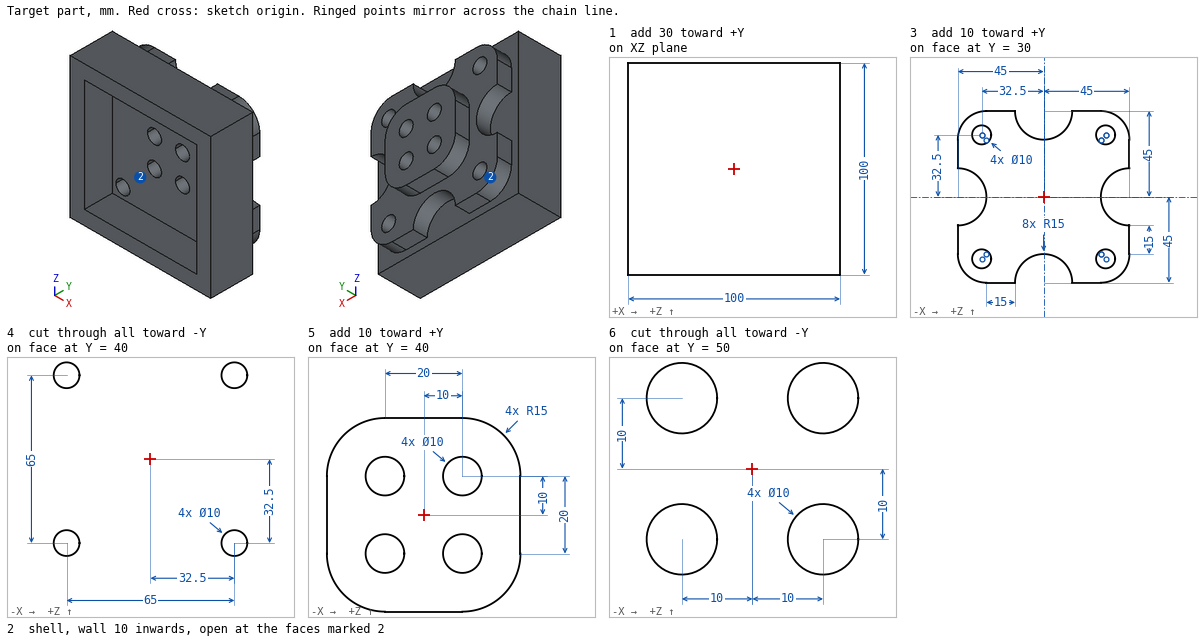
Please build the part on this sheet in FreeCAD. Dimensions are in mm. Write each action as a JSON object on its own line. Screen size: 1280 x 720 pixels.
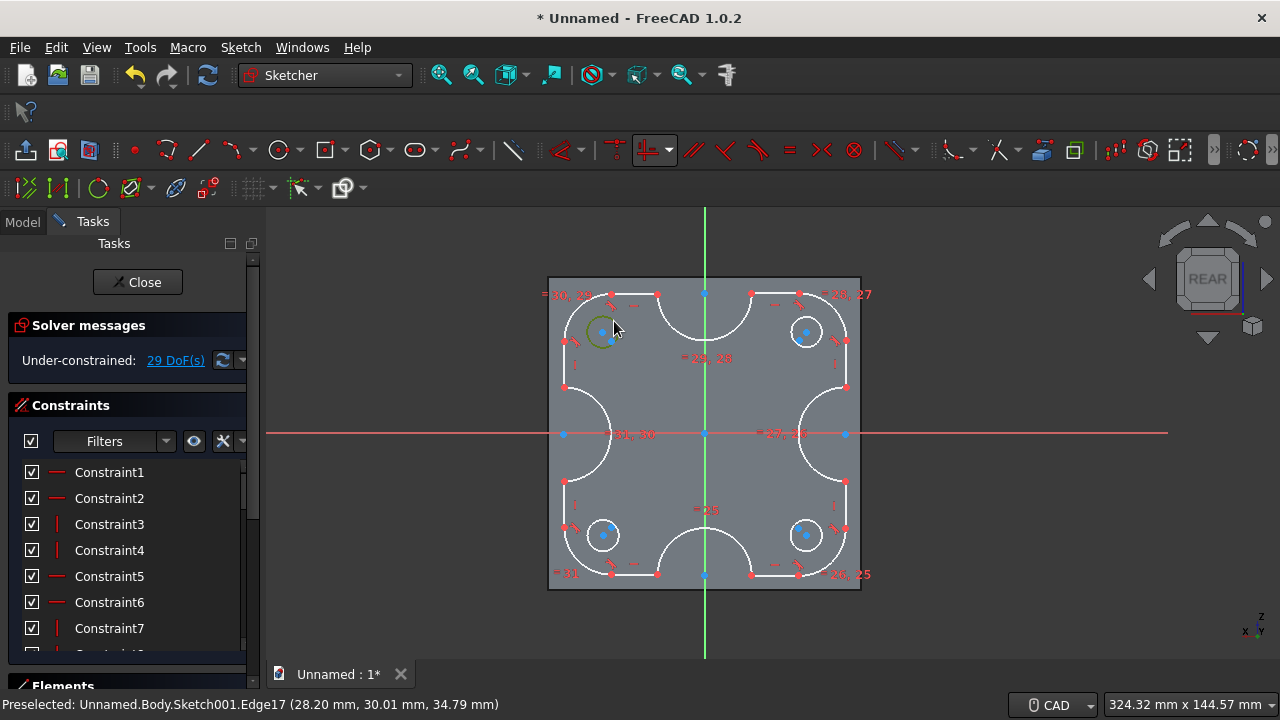
{"action": "left_click", "coordinate": [817, 321]}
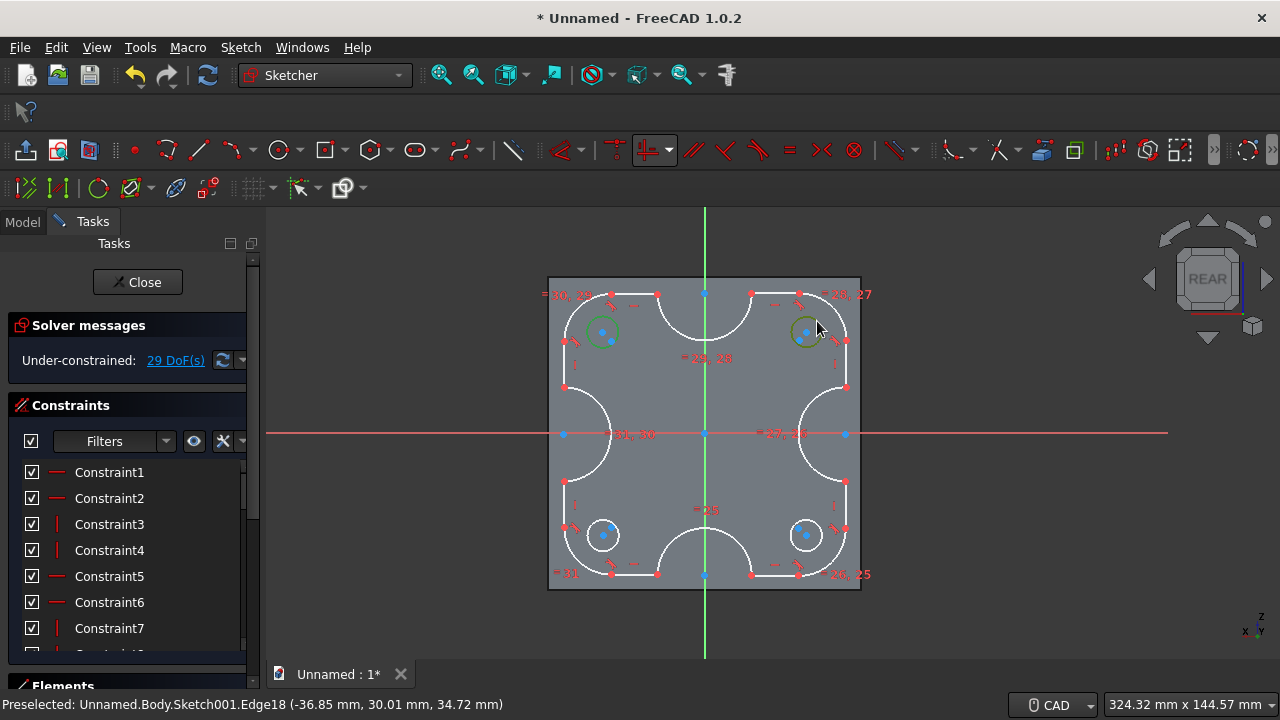
{"action": "left_click", "coordinate": [592, 525]}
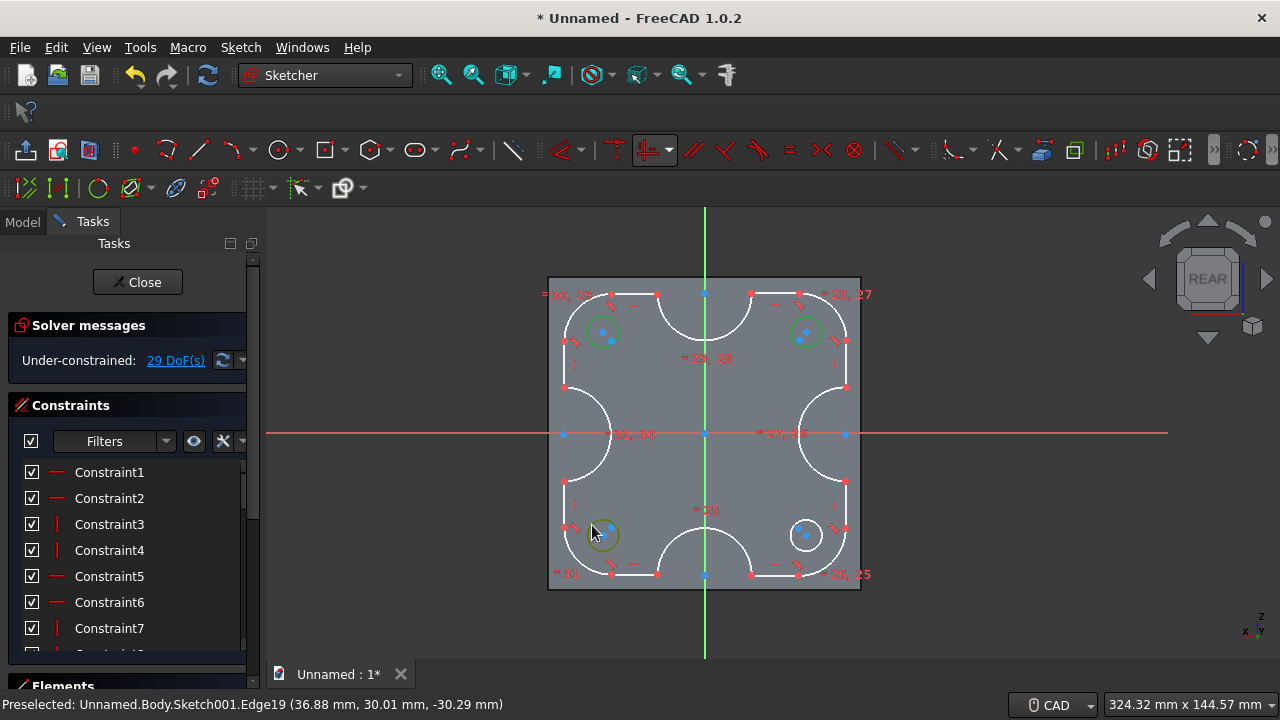
{"action": "left_click", "coordinate": [817, 524]}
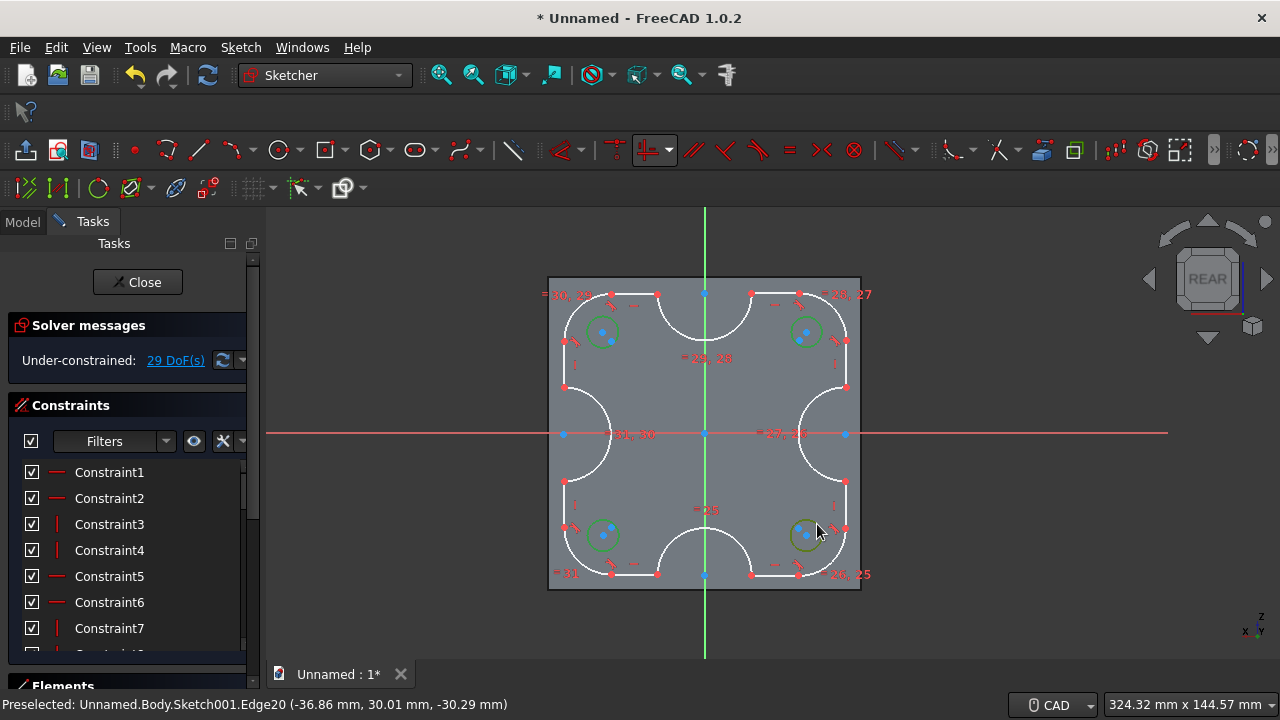
{"action": "left_click", "coordinate": [790, 150]}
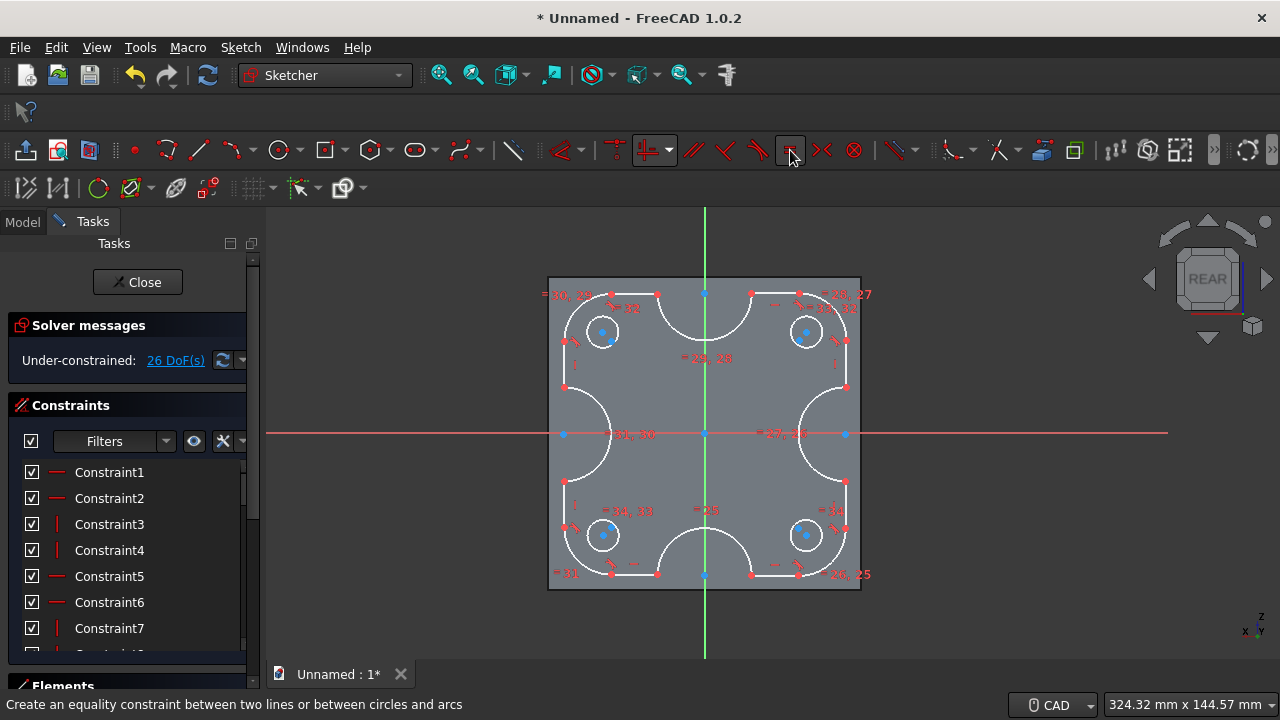
{"action": "left_click", "coordinate": [705, 575]}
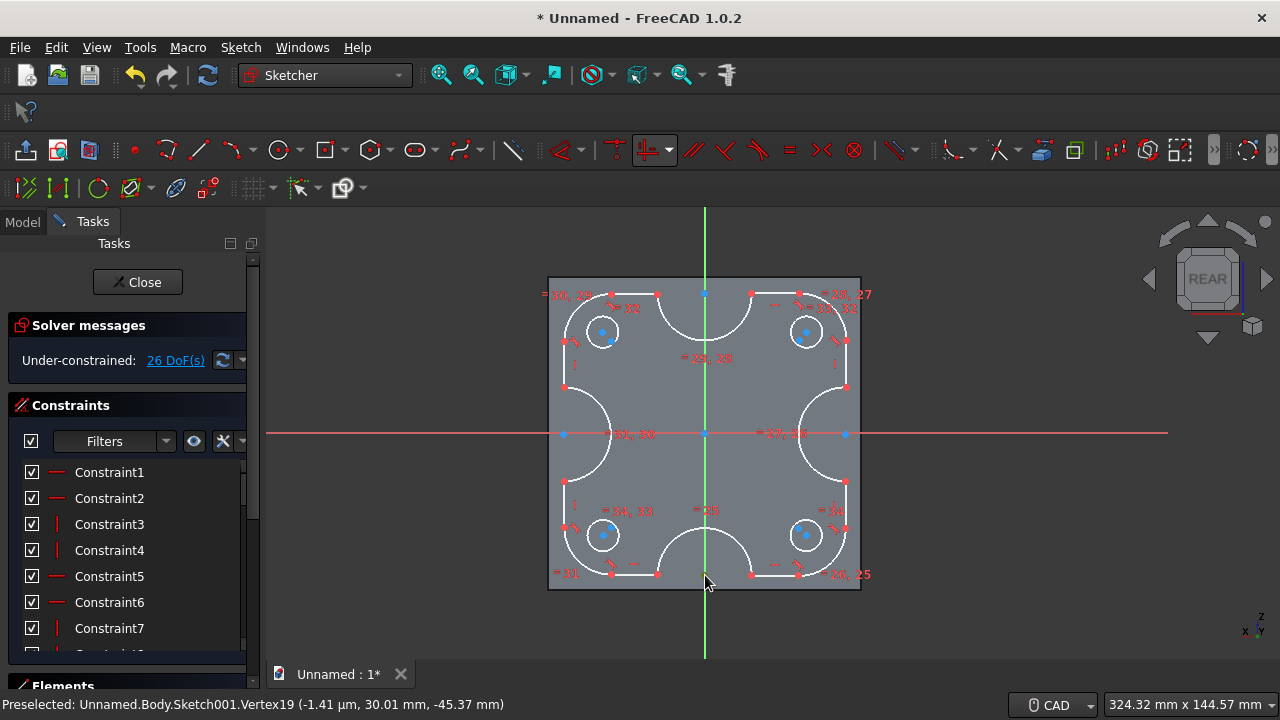
{"action": "left_click", "coordinate": [705, 603]}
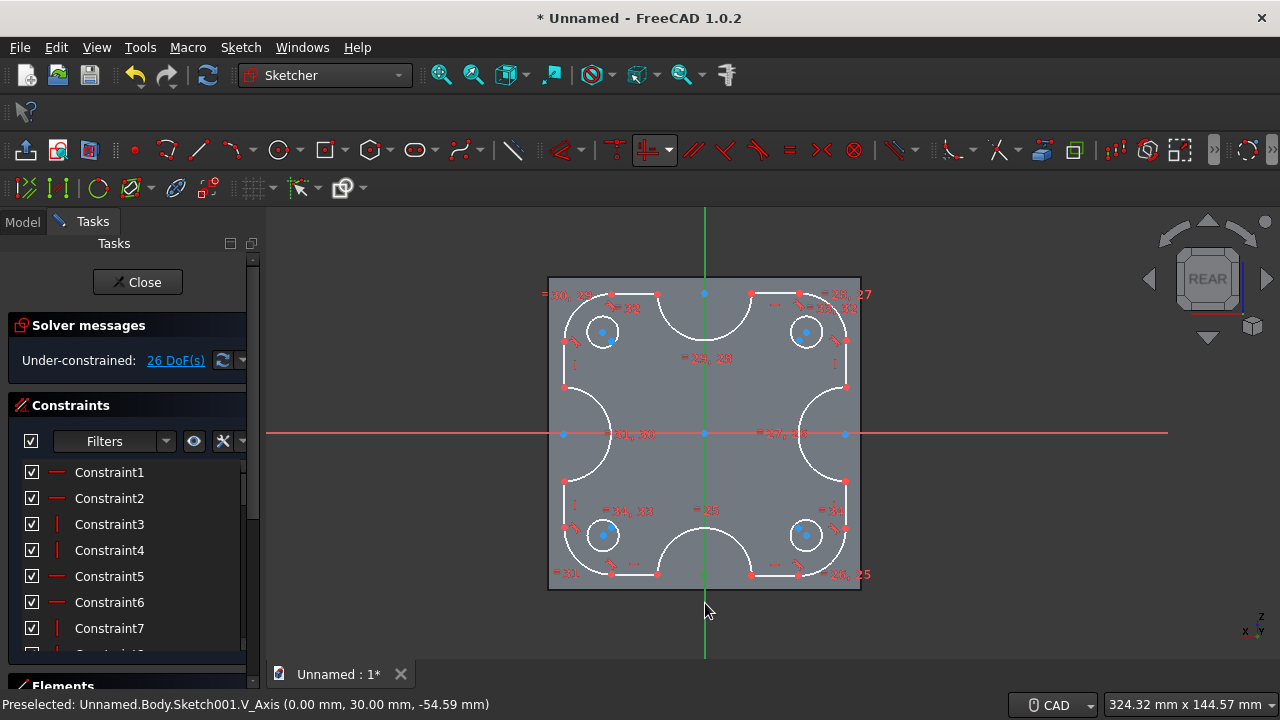
{"action": "left_click", "coordinate": [616, 150]}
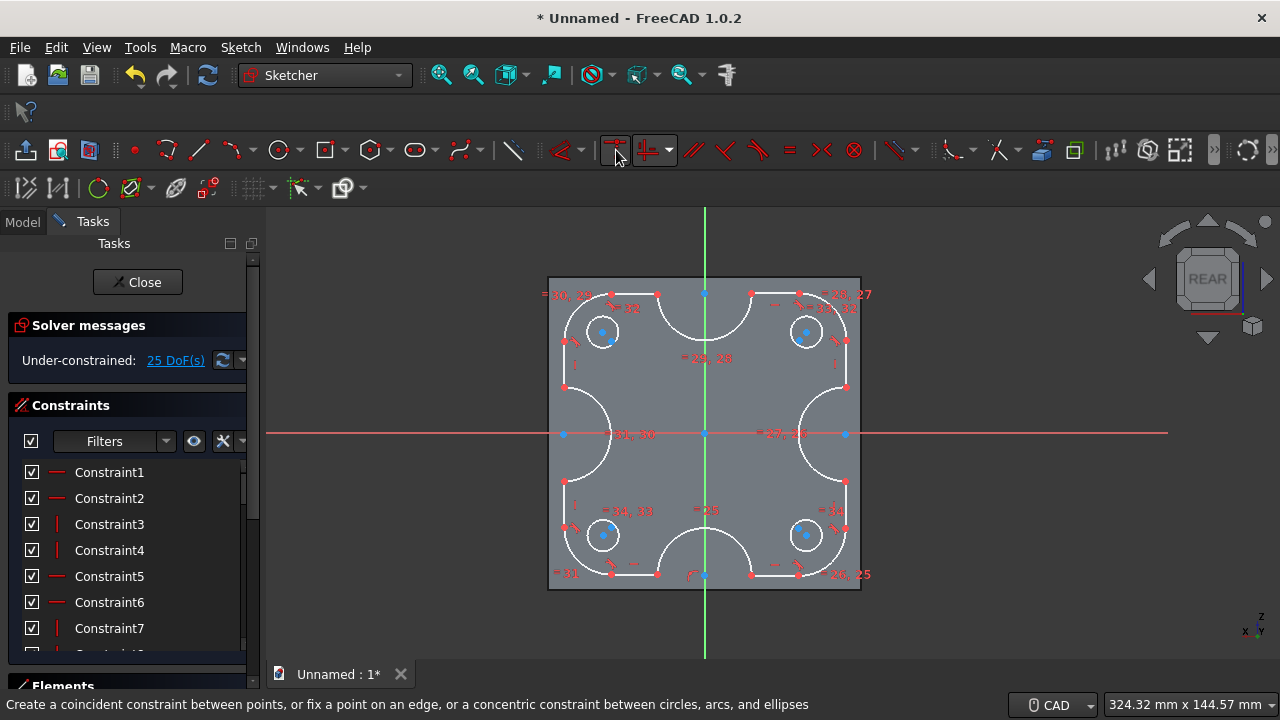
{"action": "left_click", "coordinate": [846, 434]}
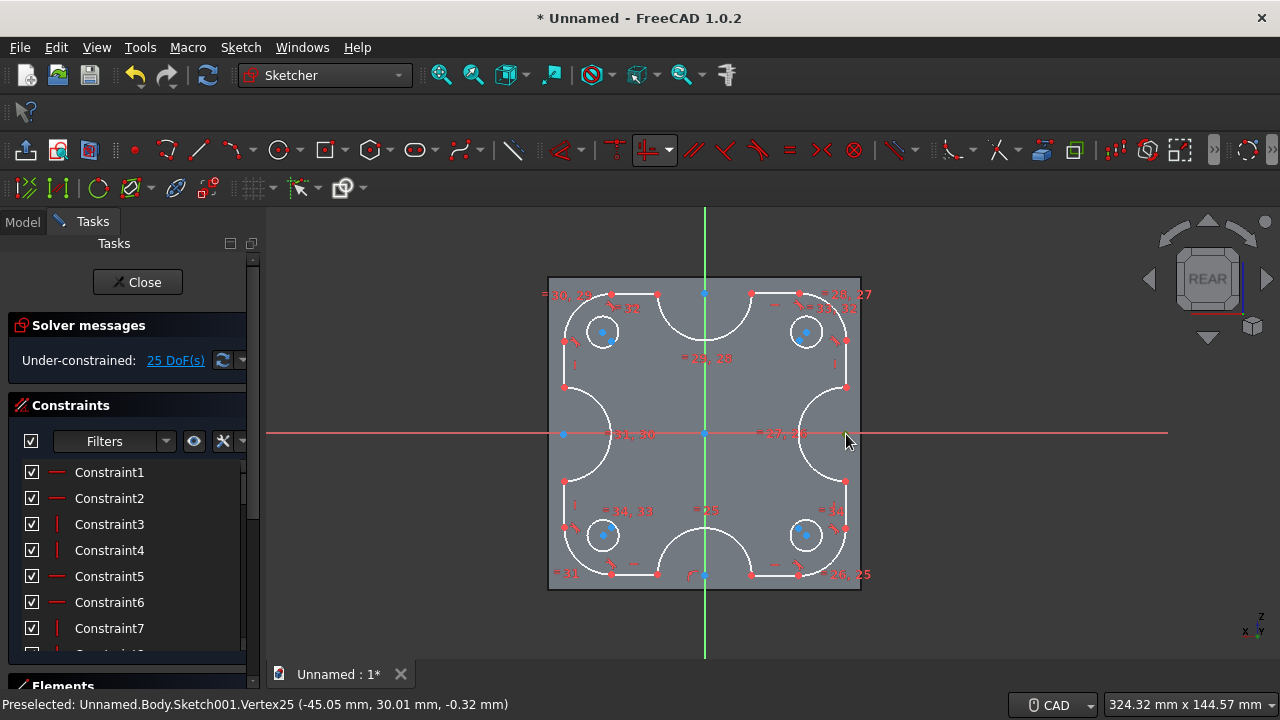
{"action": "left_click", "coordinate": [353, 433]}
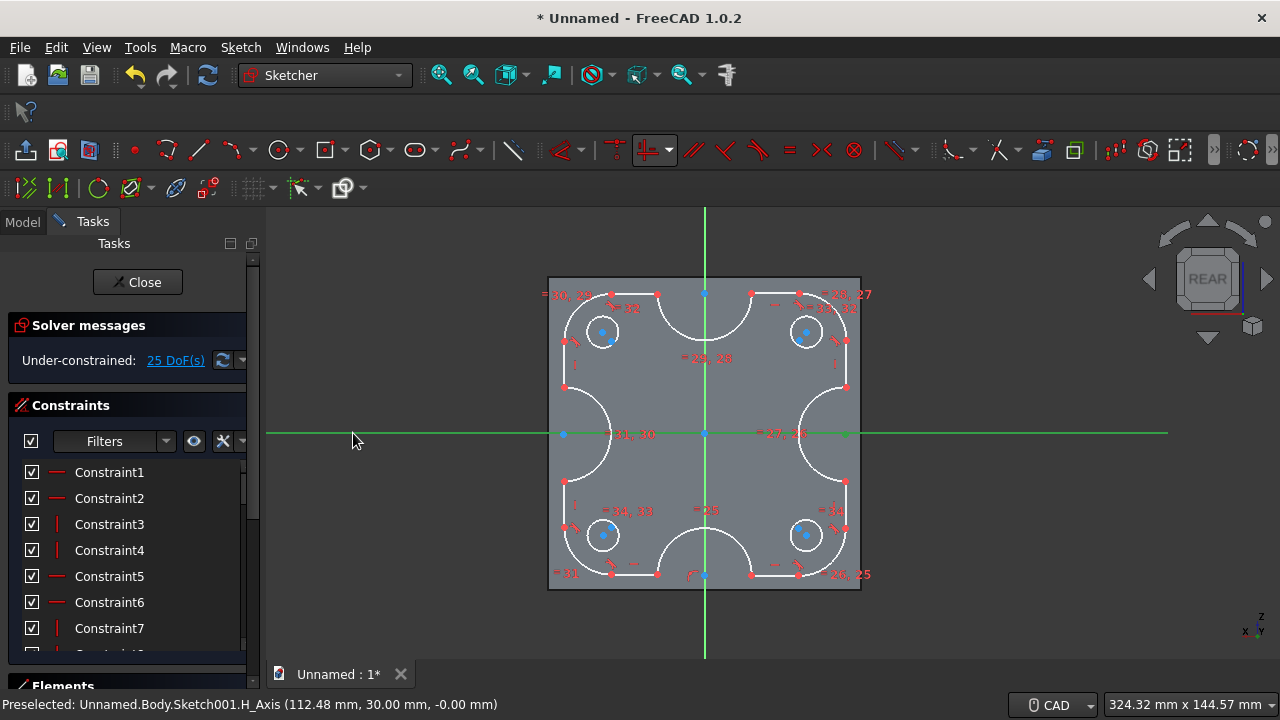
{"action": "left_click", "coordinate": [616, 150]}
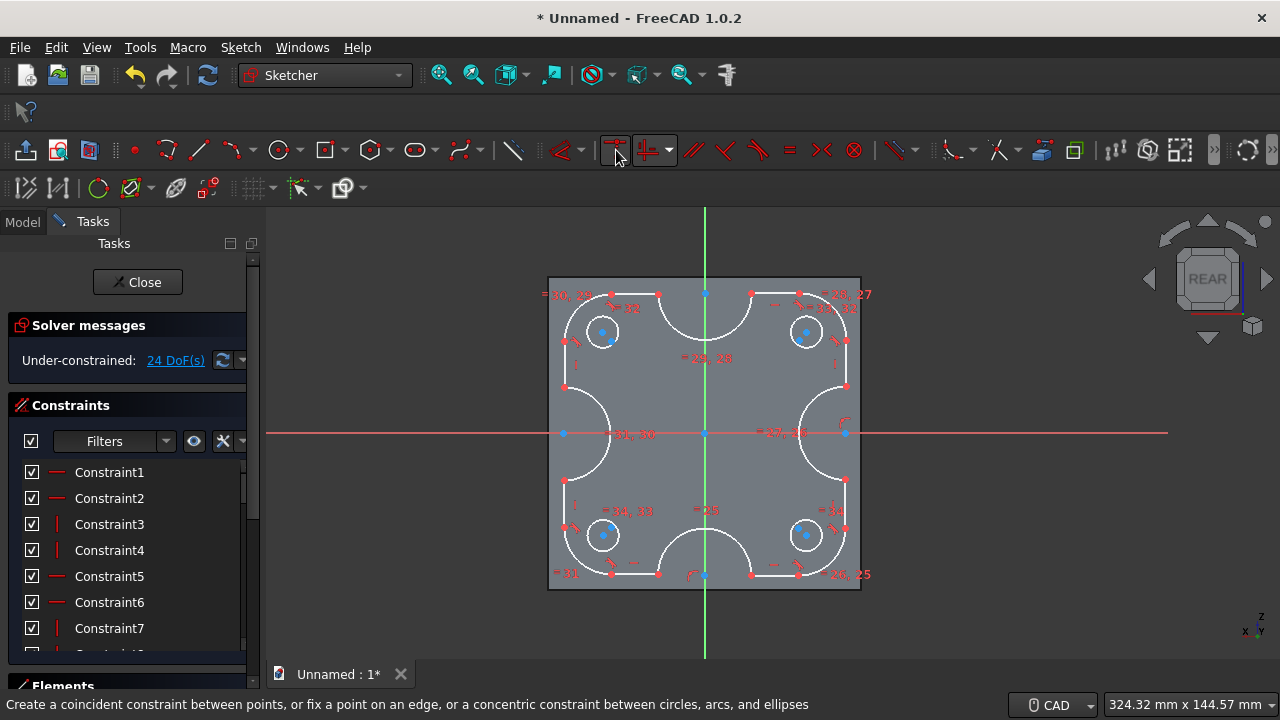
{"action": "left_click", "coordinate": [705, 293]}